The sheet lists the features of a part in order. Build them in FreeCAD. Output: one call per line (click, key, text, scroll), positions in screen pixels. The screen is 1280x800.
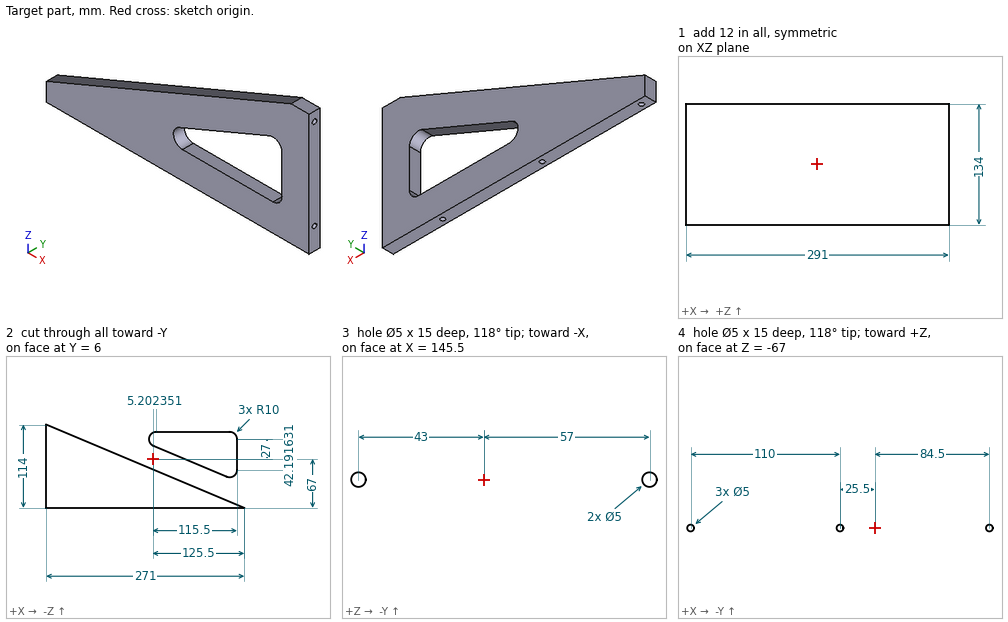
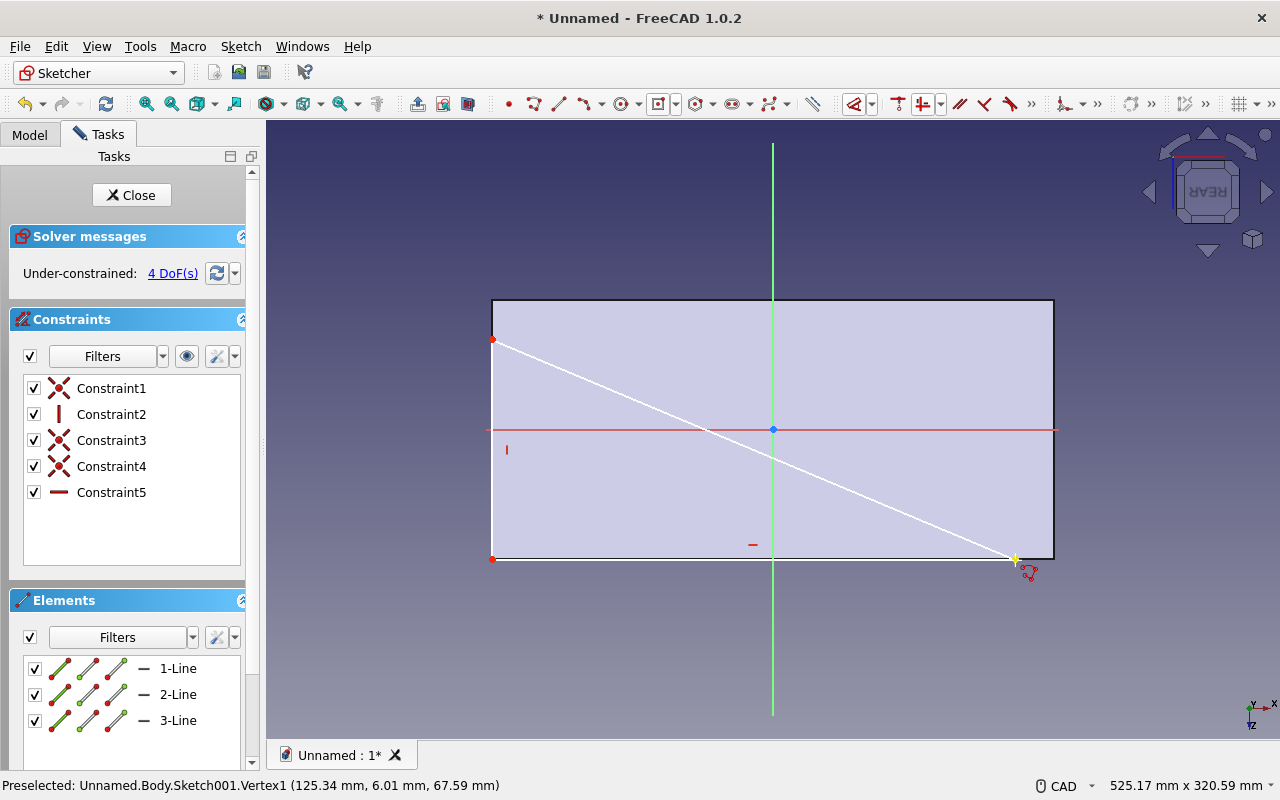
click(559, 104)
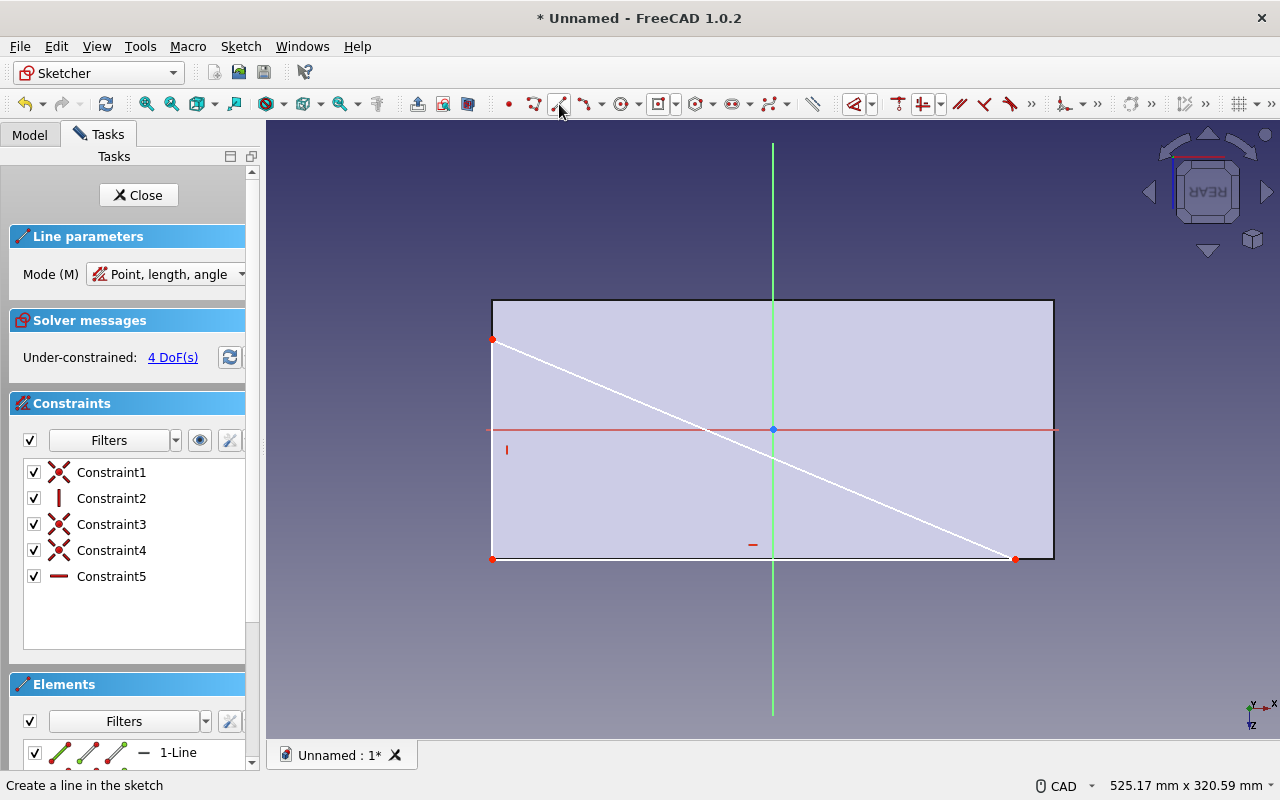
click(996, 459)
click(996, 377)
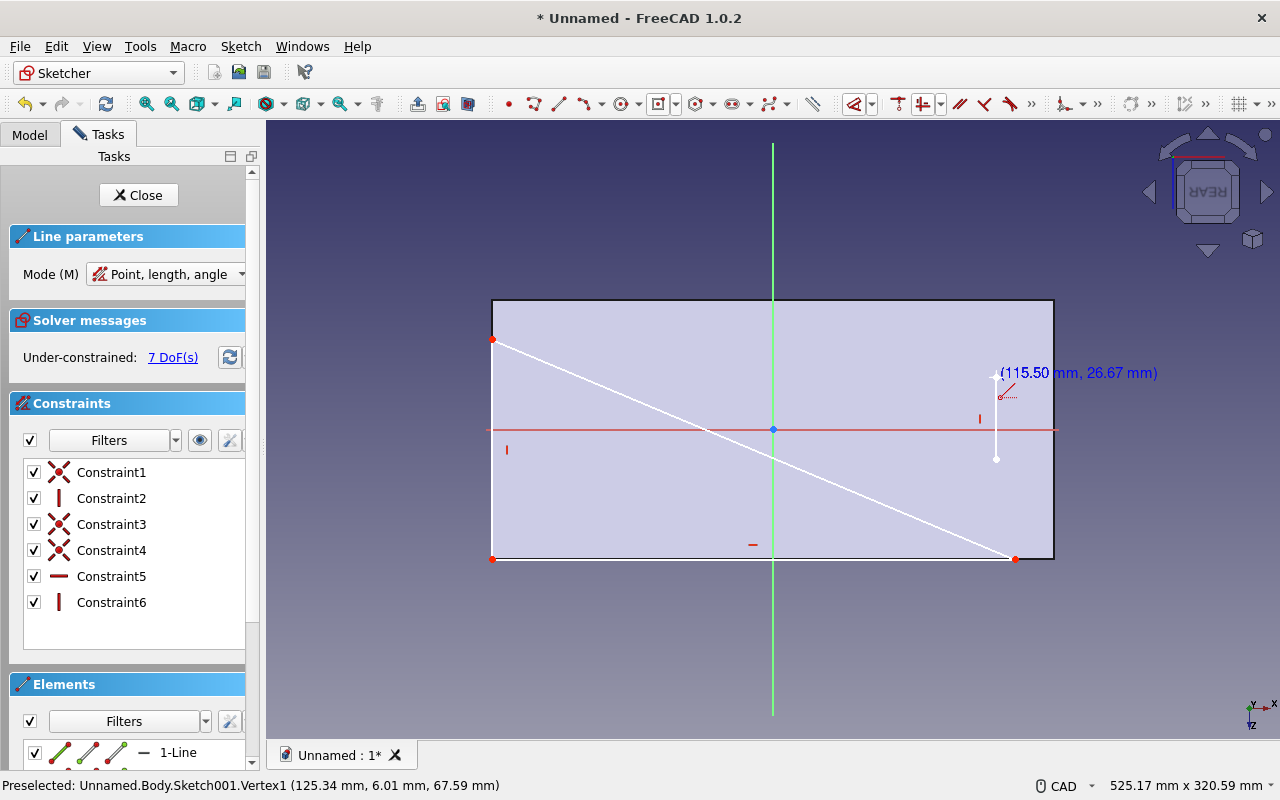
click(977, 358)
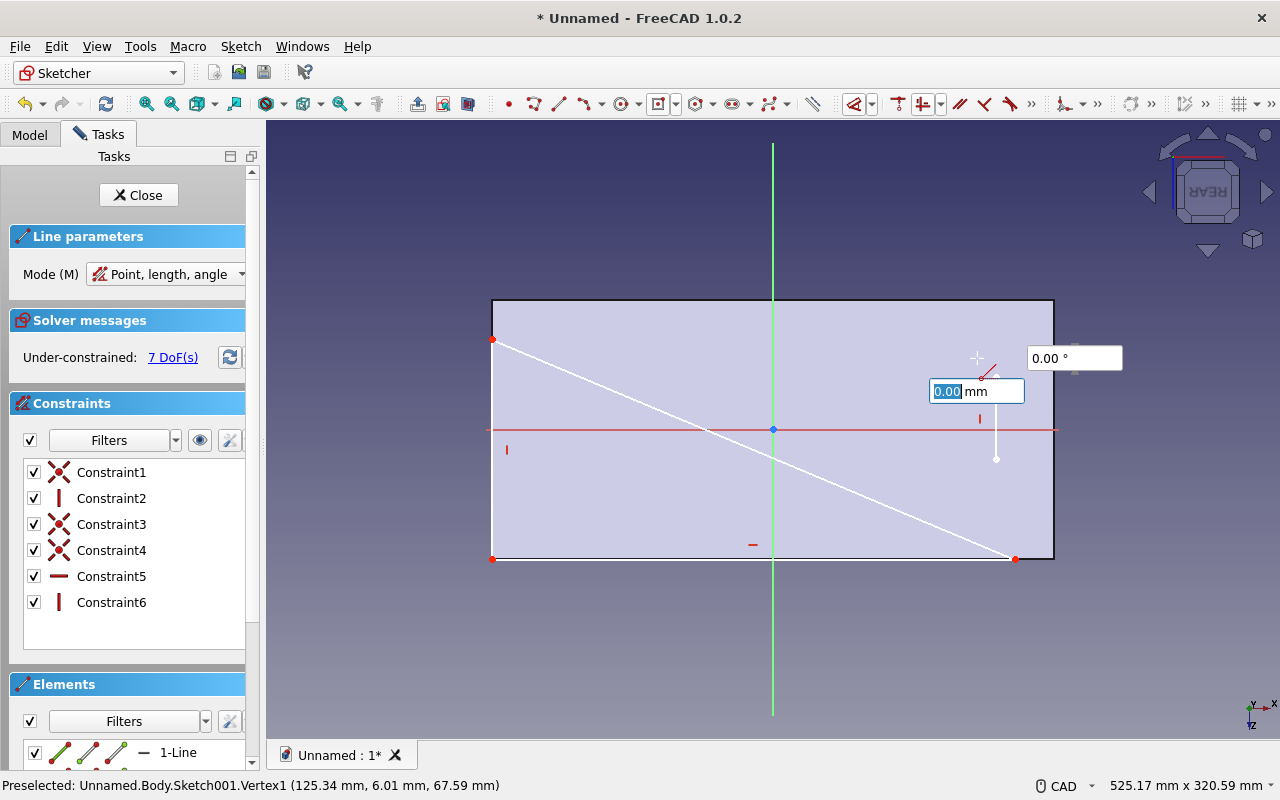
scroll(783, 358, up, 3)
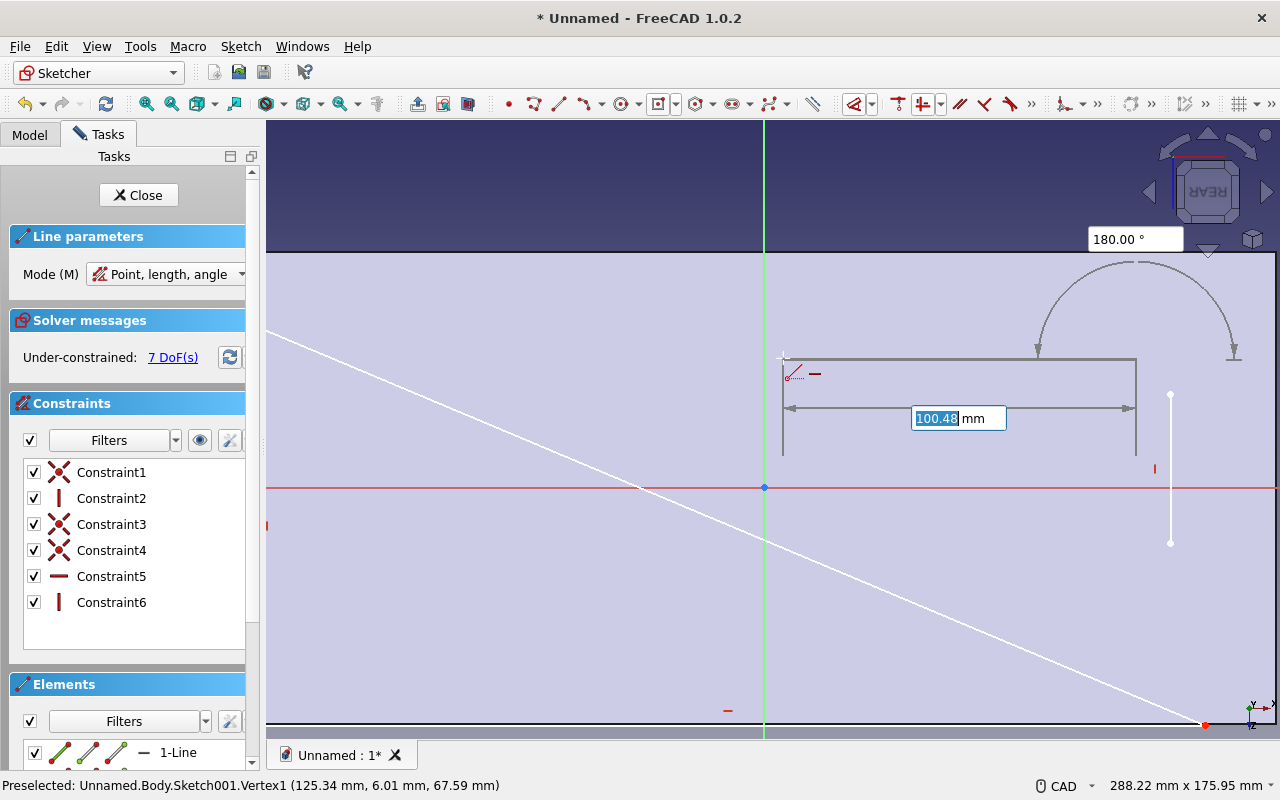
click(783, 358)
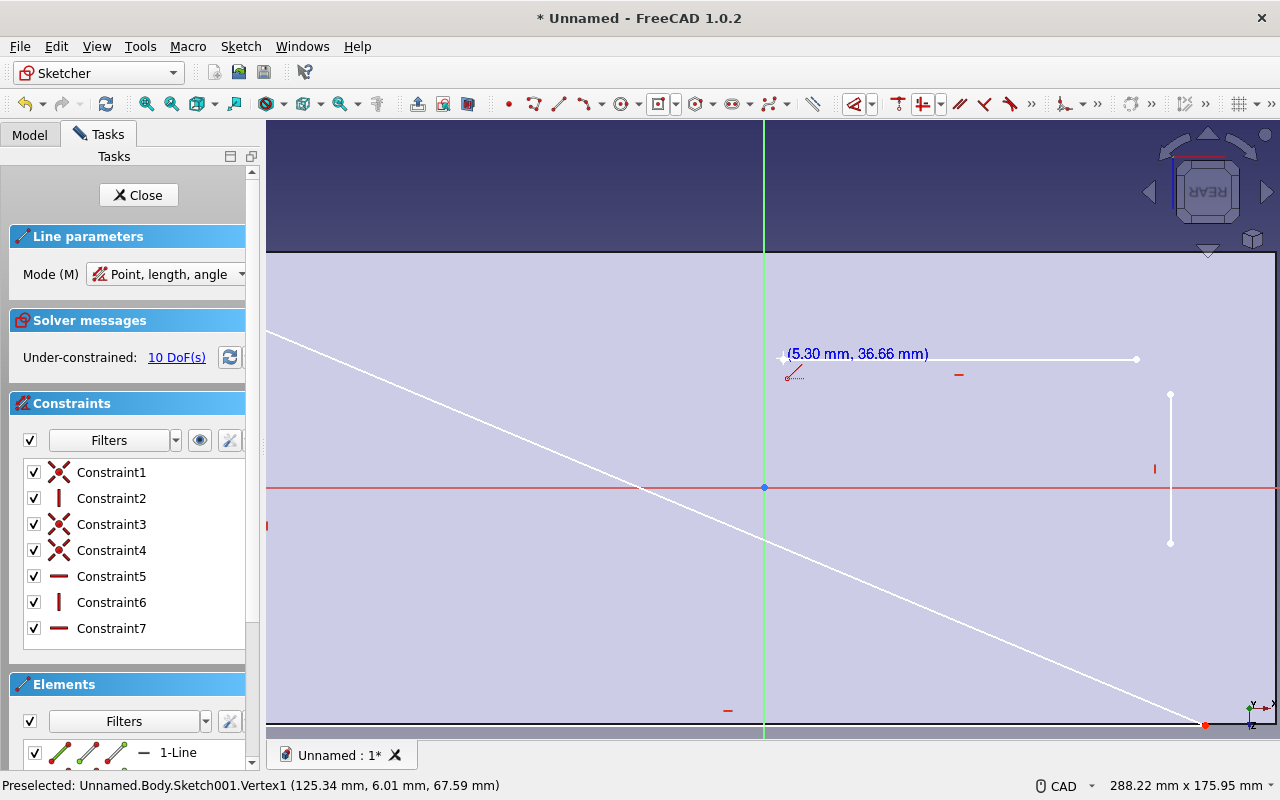
scroll(769, 425, up, 7)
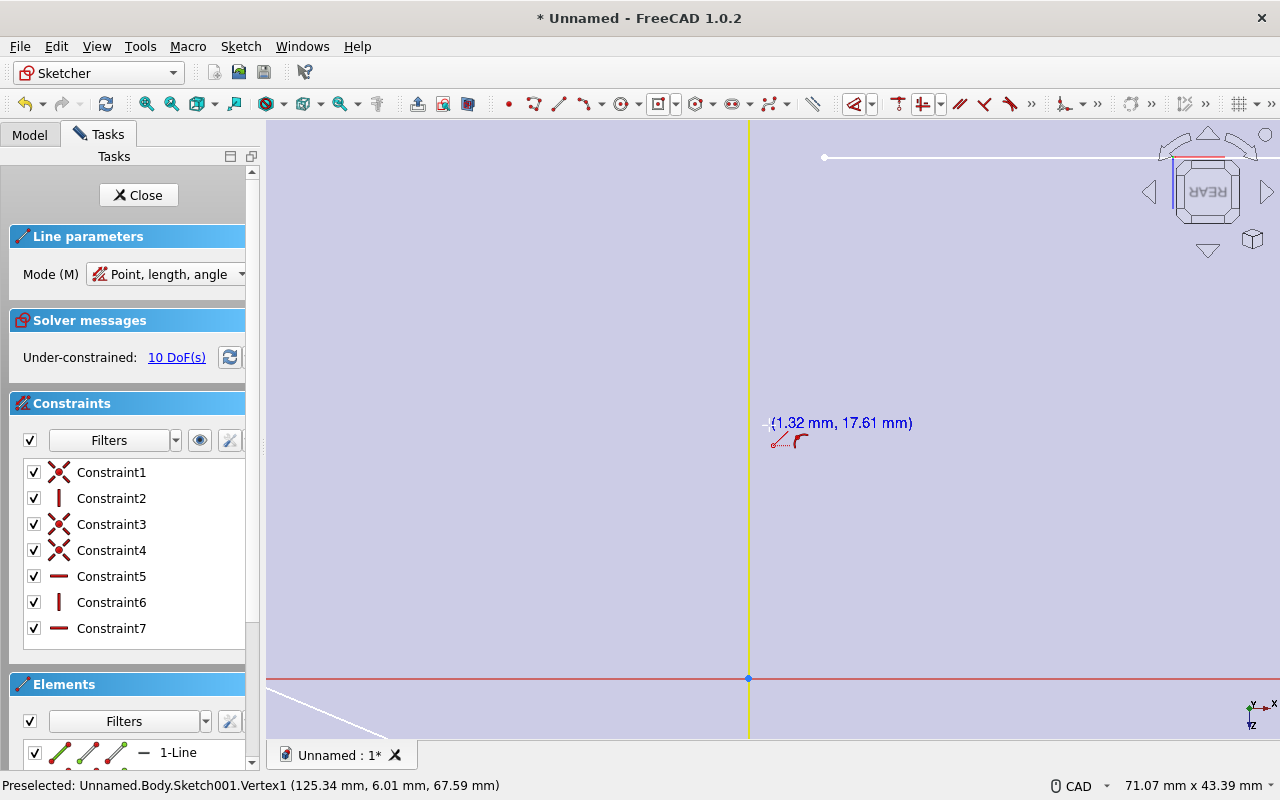
click(768, 425)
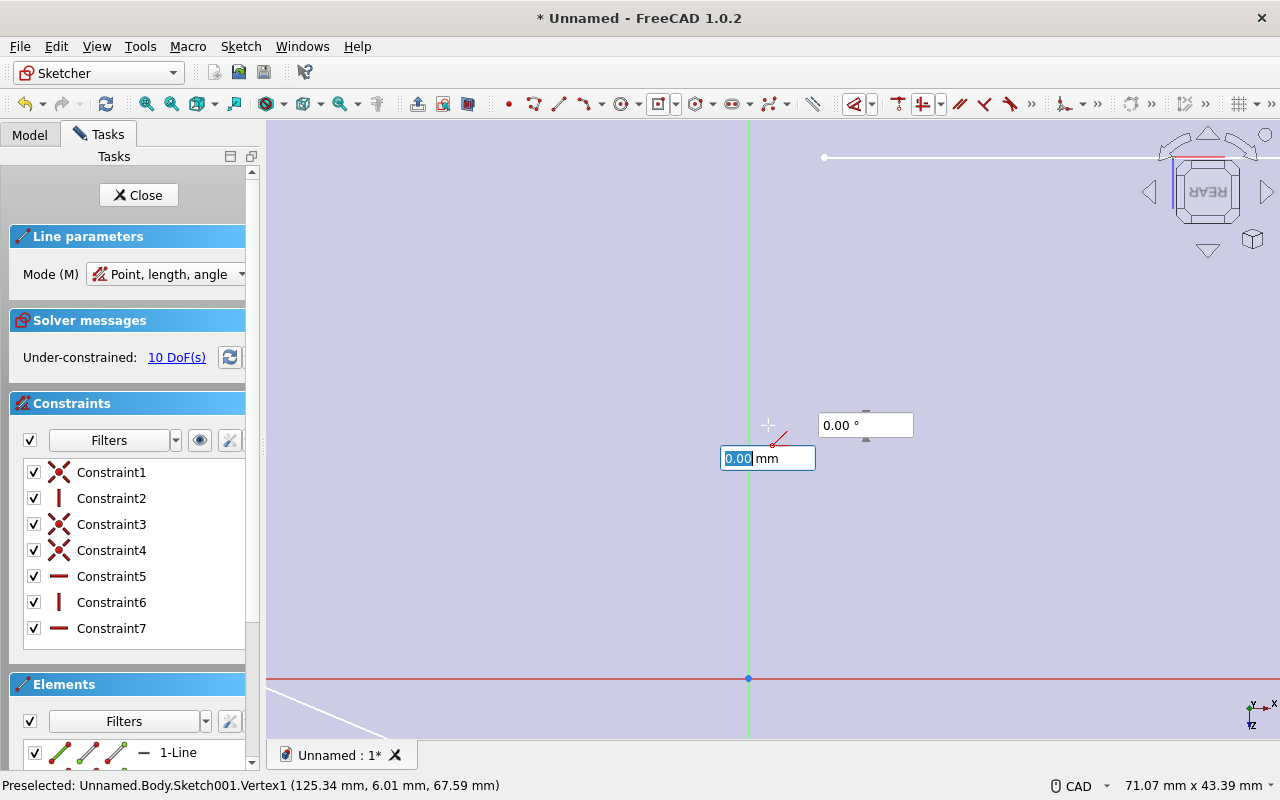
scroll(724, 352, down, 9)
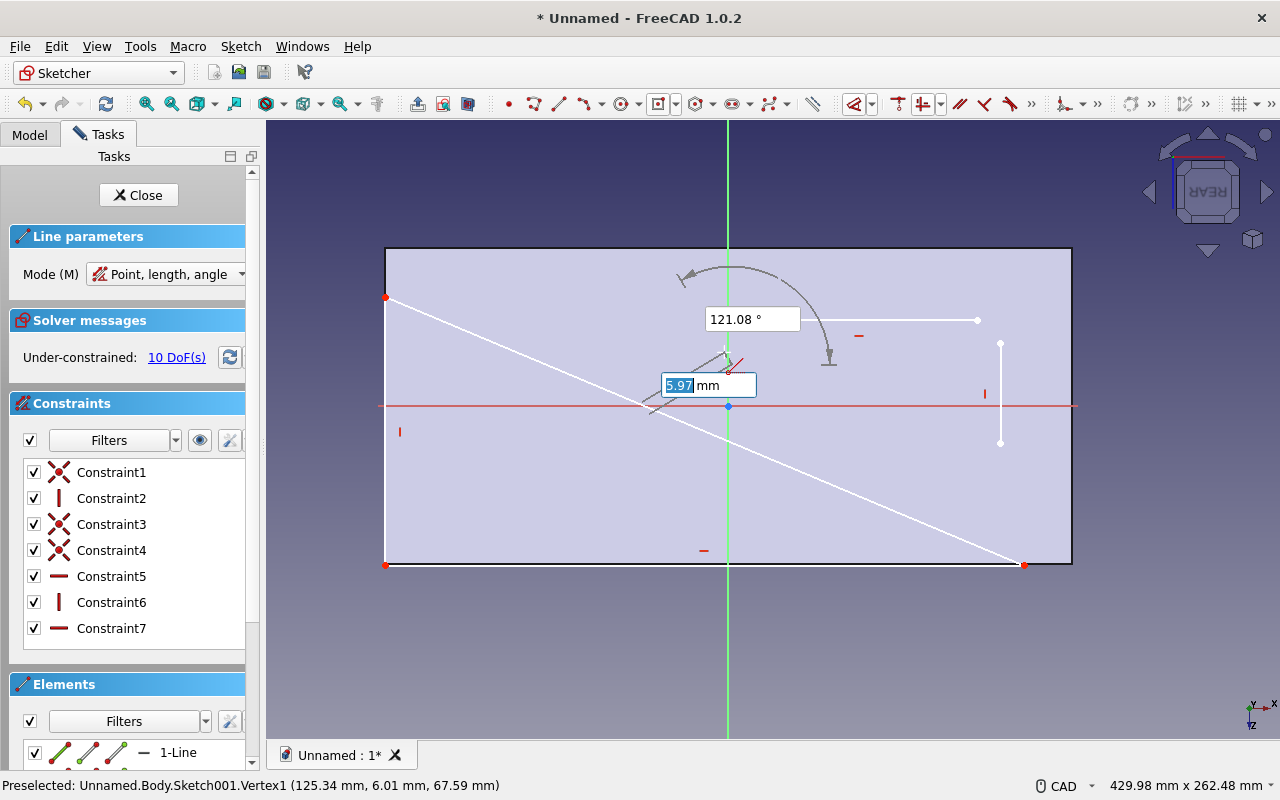
click(968, 464)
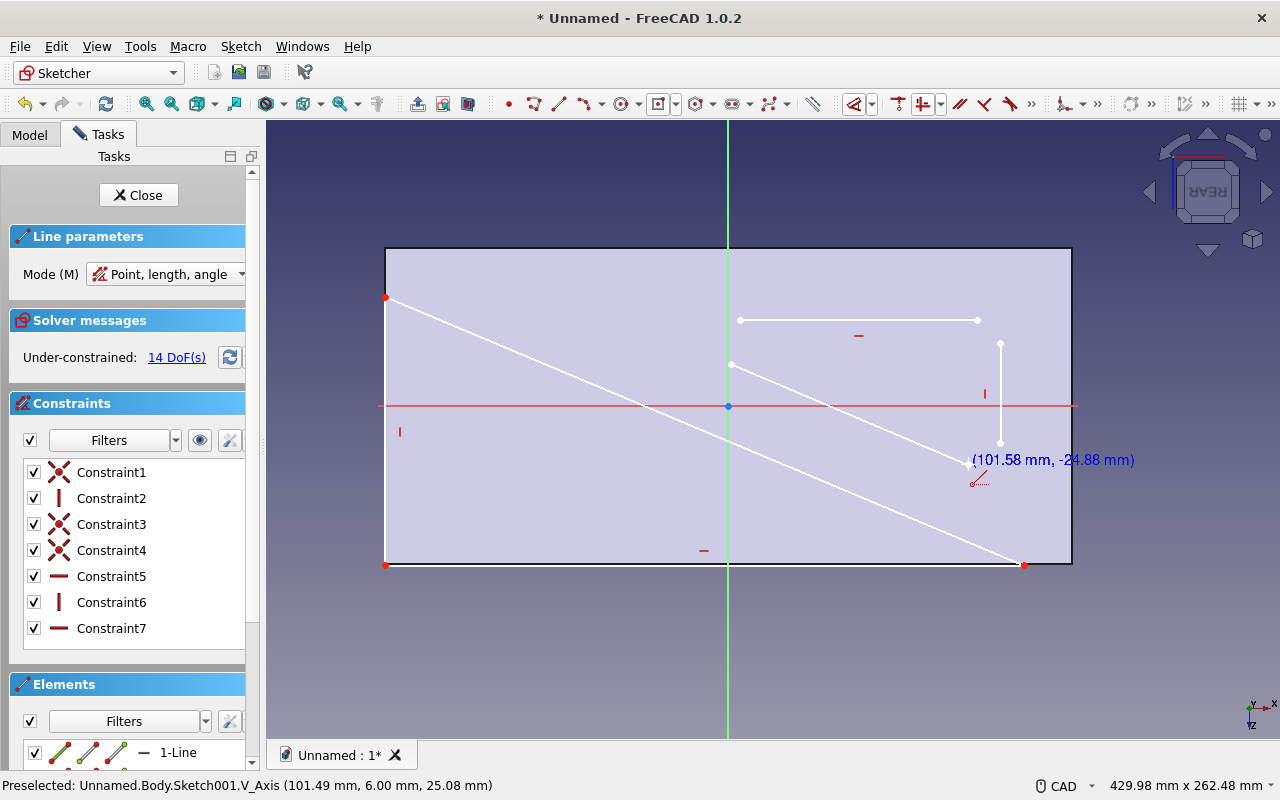
click(584, 104)